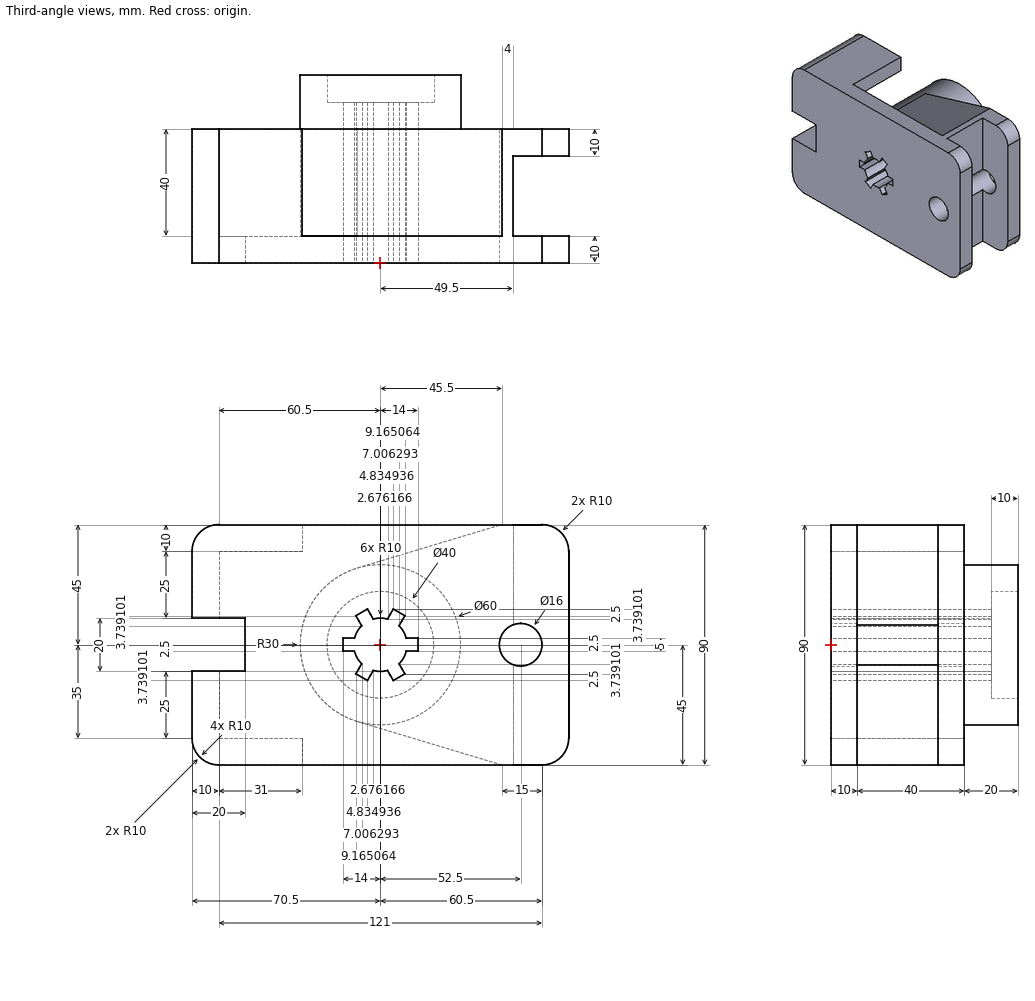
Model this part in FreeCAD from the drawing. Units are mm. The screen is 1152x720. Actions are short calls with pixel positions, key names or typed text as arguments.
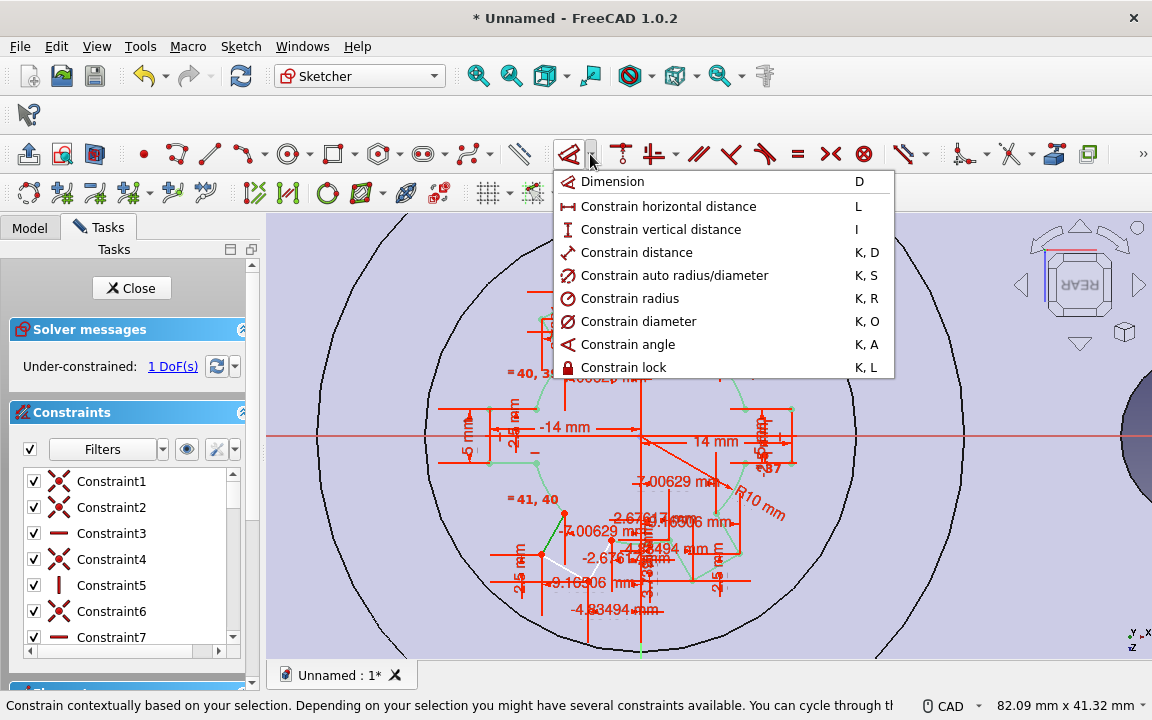
click(724, 230)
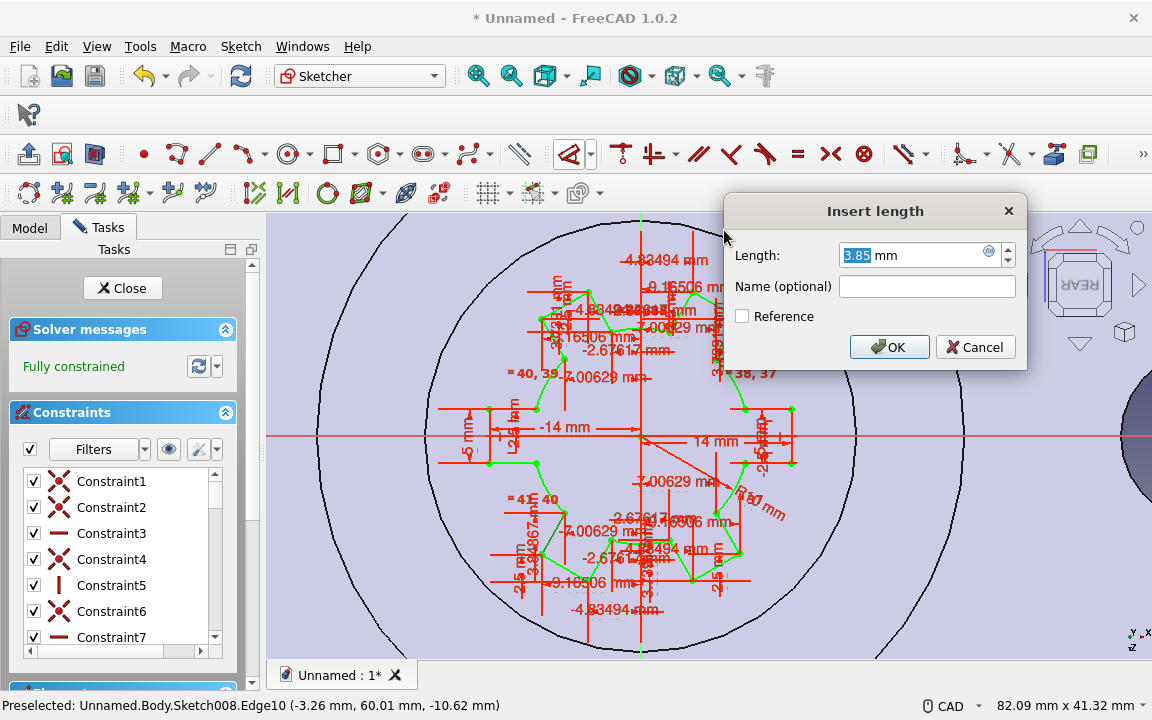
text(3.739101)
key(Return)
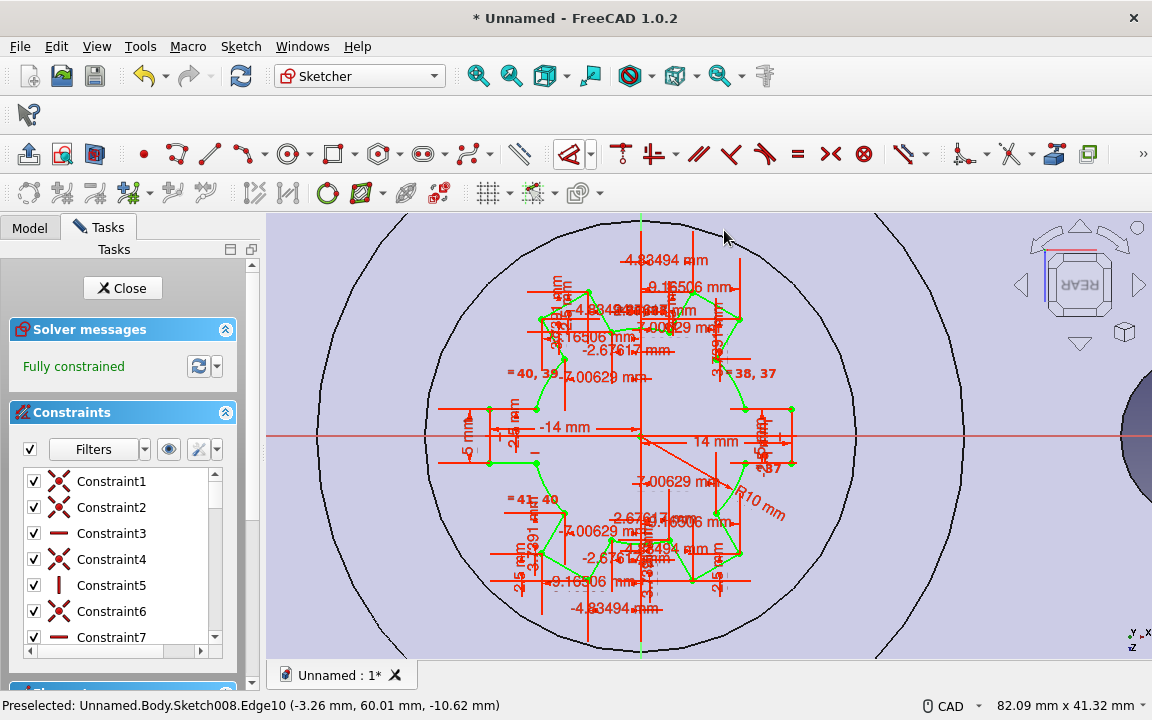
click(123, 288)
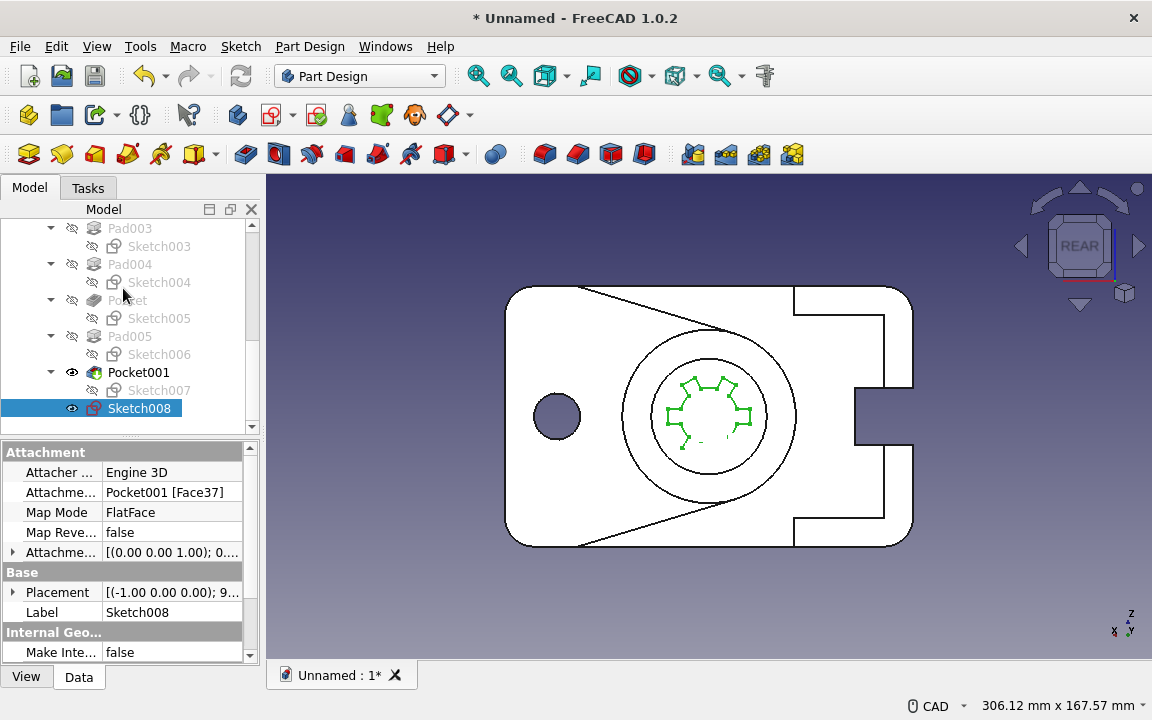
click(246, 154)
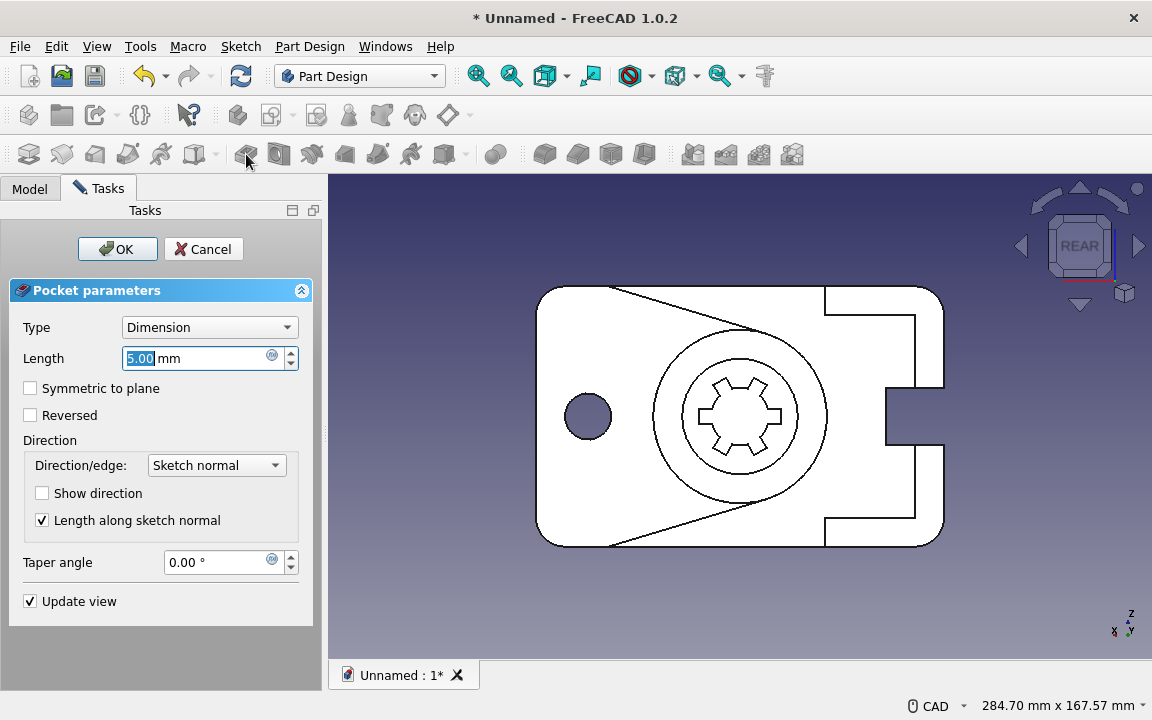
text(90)
key(Tab)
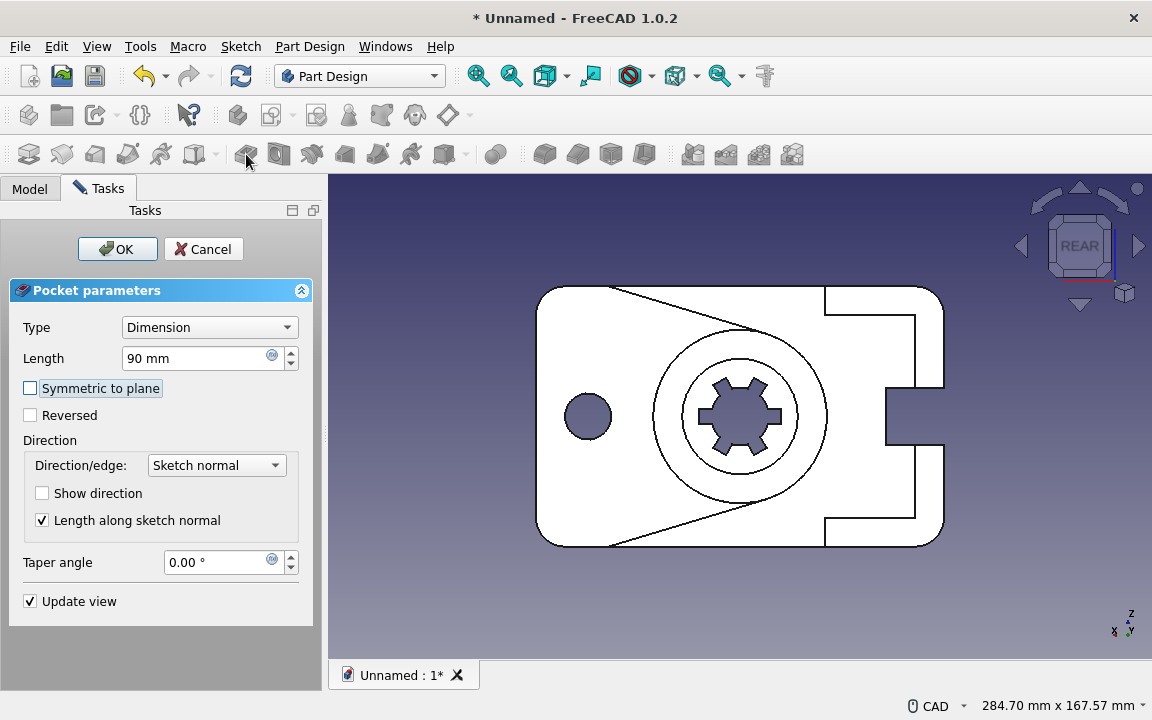
click(118, 249)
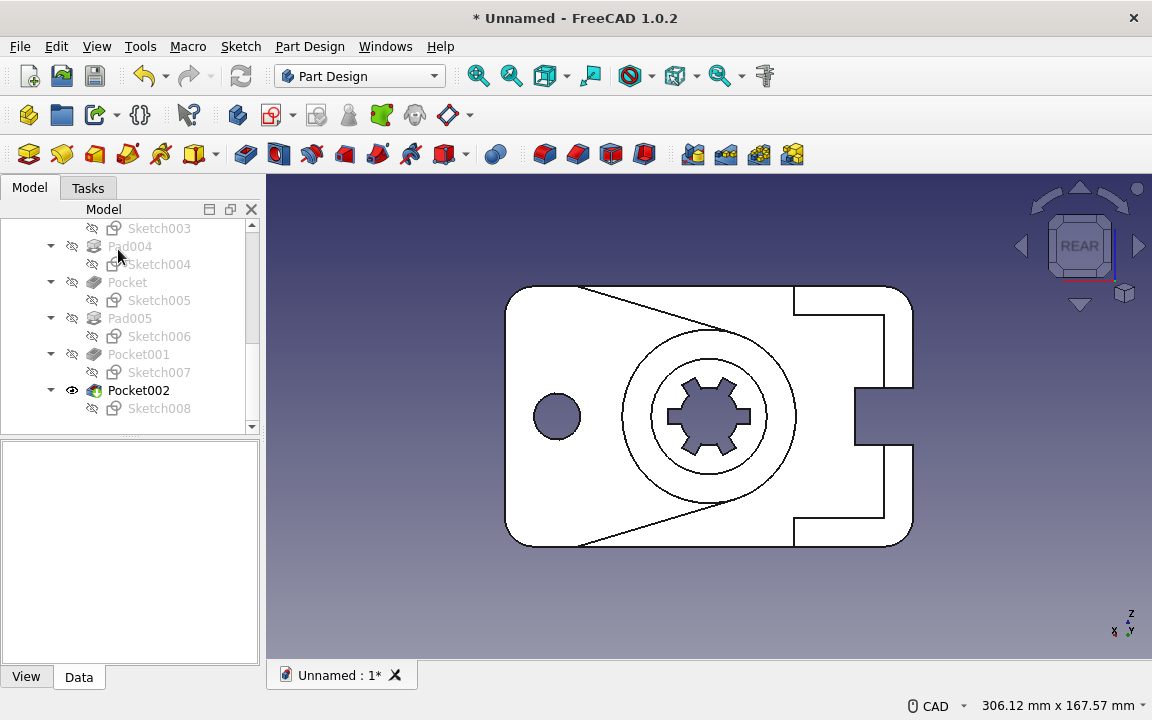
key(0)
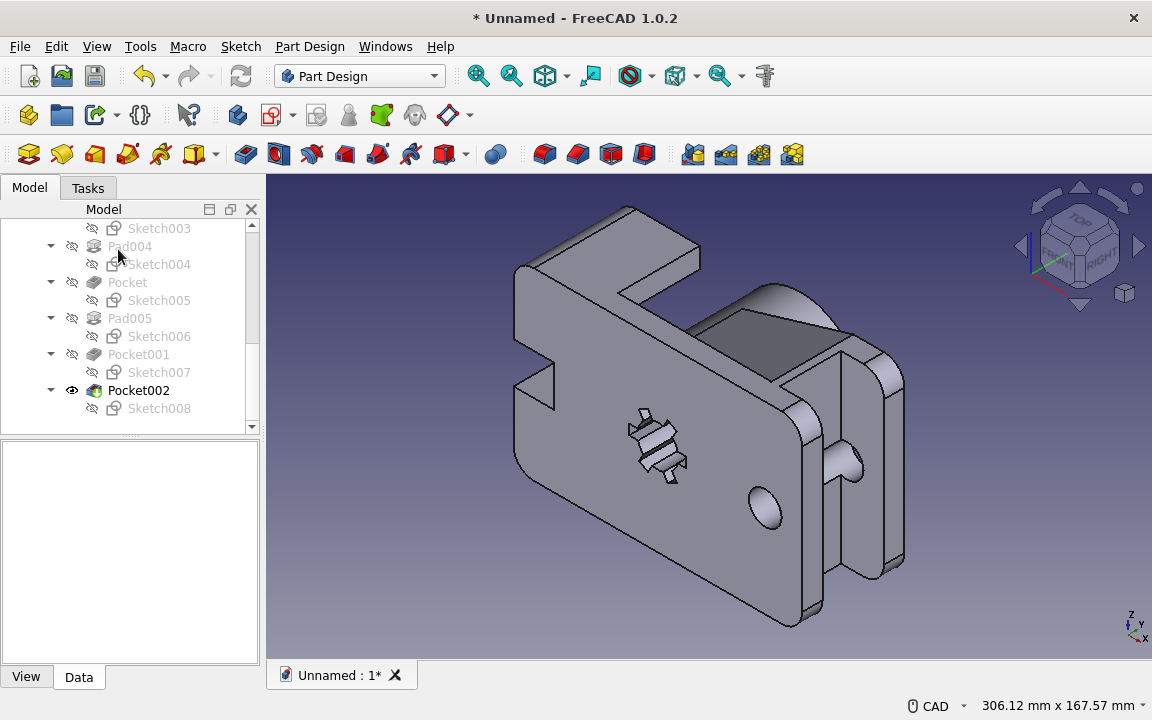
click(479, 76)